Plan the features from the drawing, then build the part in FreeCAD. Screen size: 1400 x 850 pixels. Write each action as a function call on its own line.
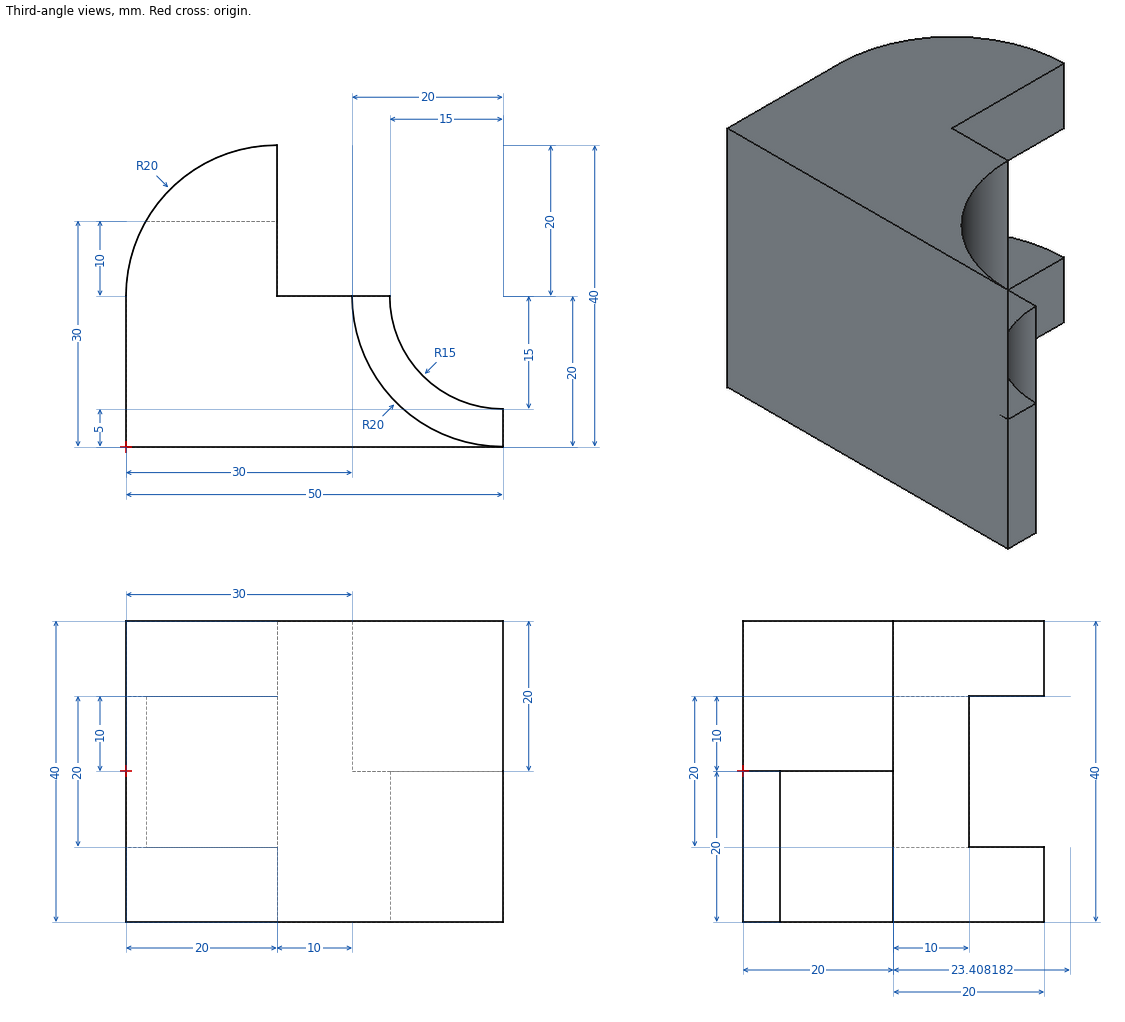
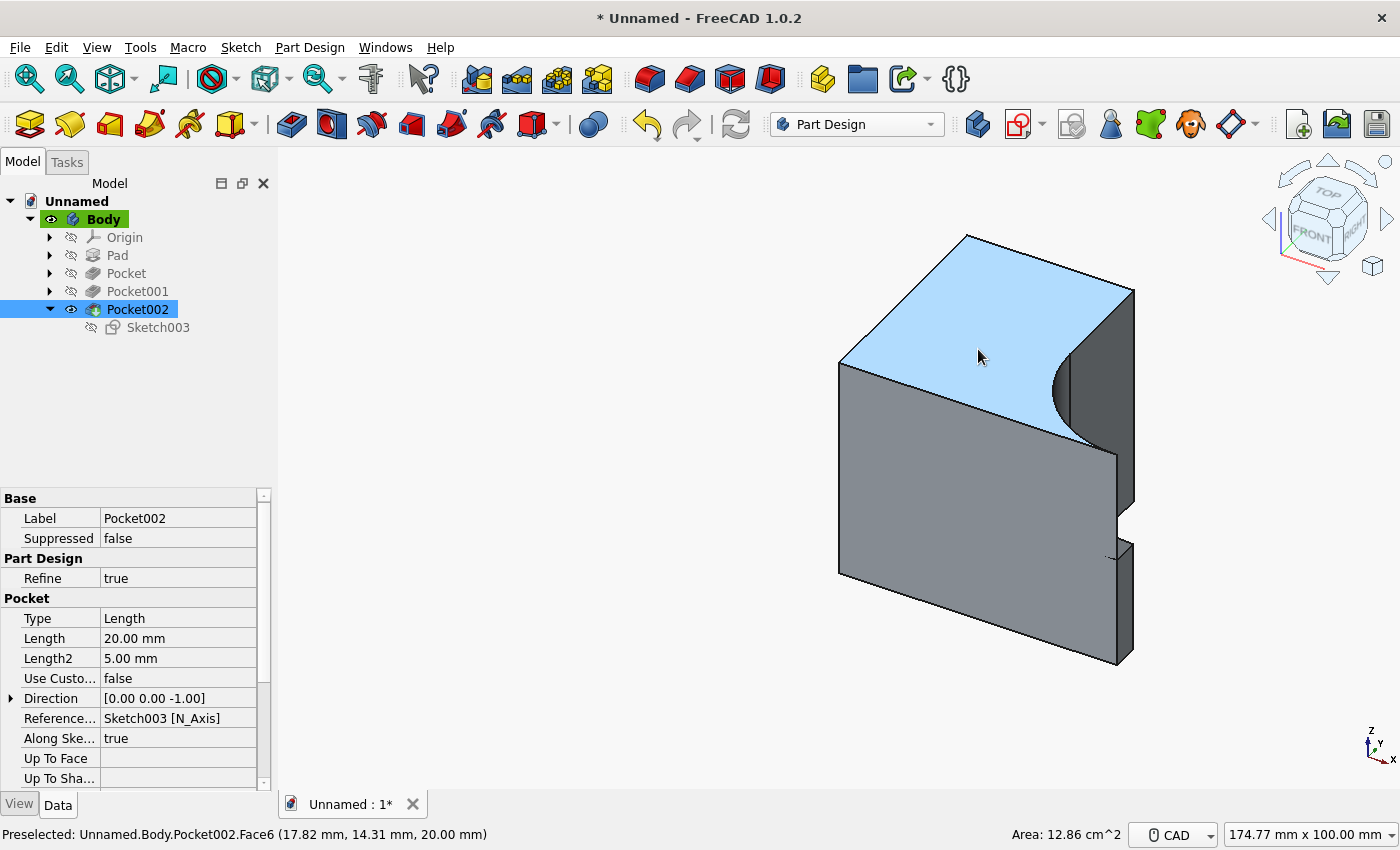
click(1018, 124)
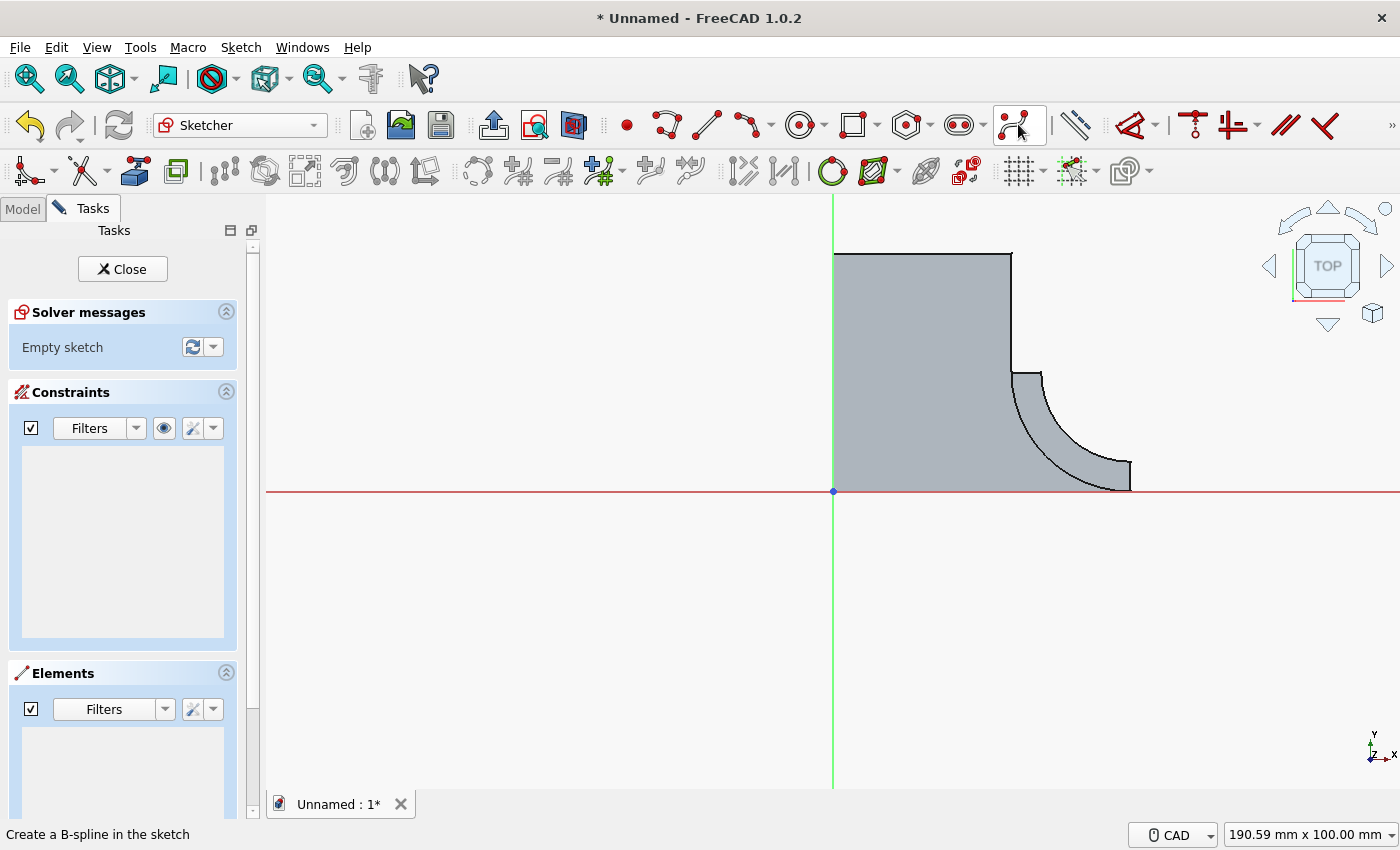
scroll(1153, 222, up, 2)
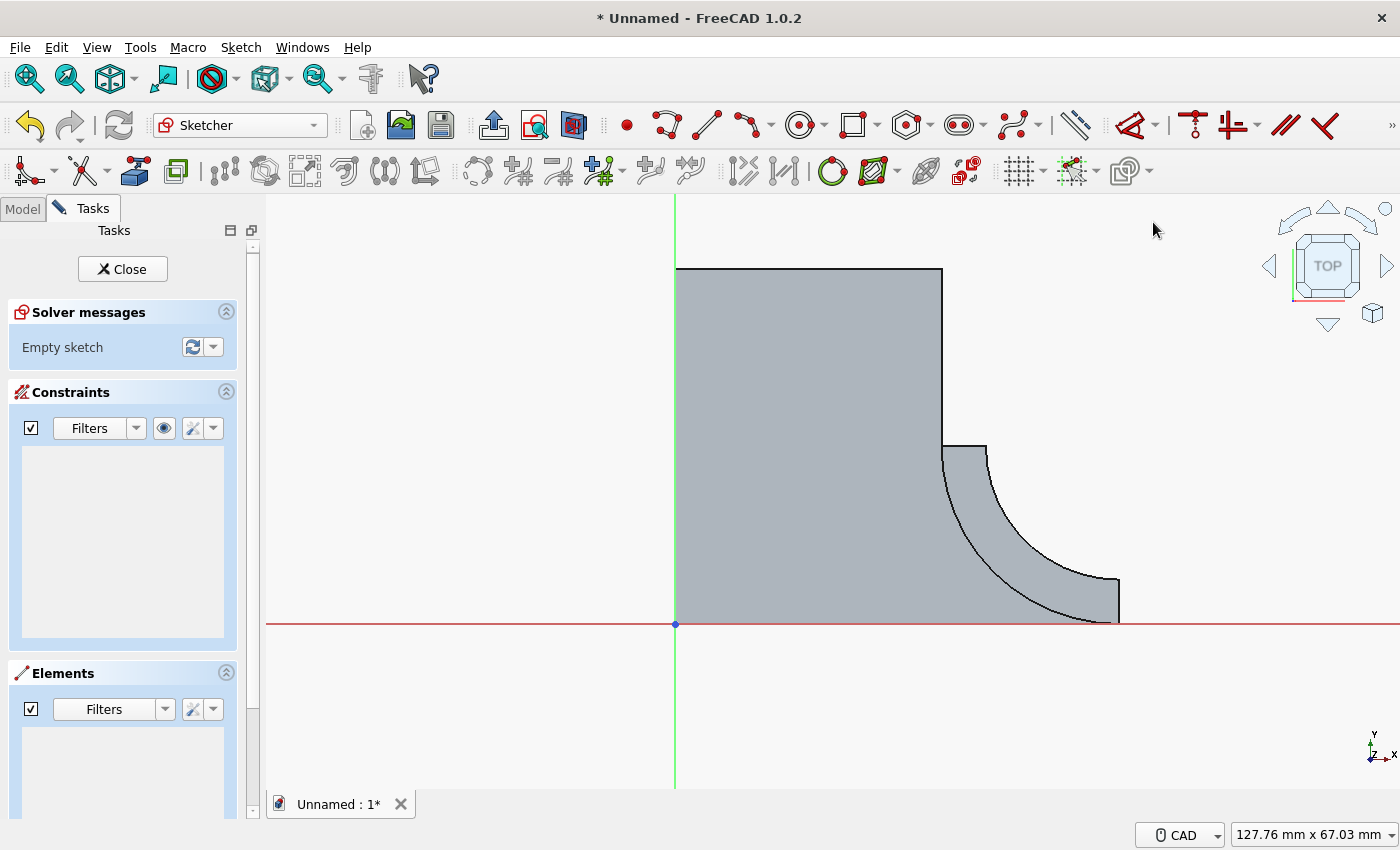
click(668, 126)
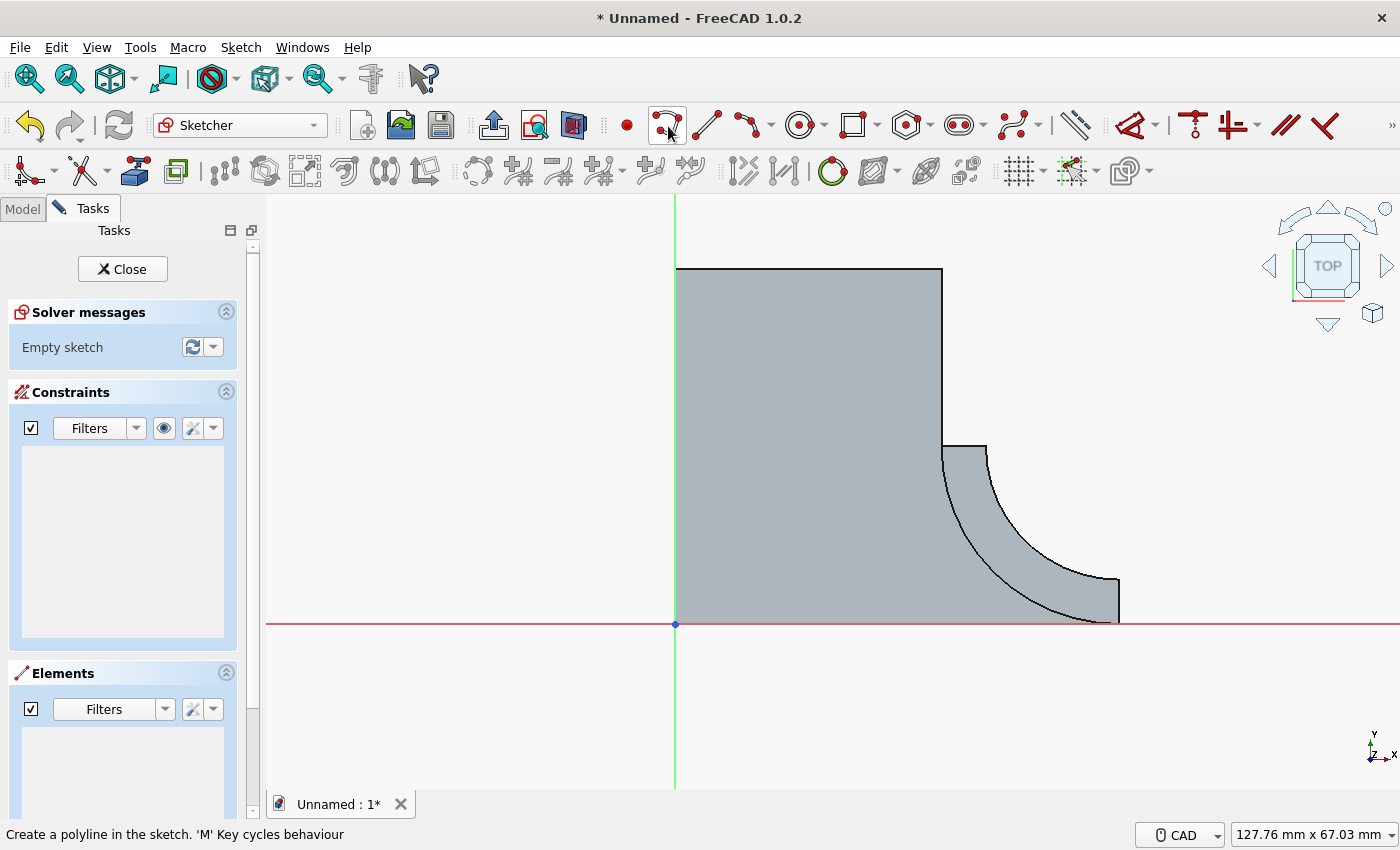
click(853, 269)
click(675, 269)
click(684, 446)
right_click(684, 446)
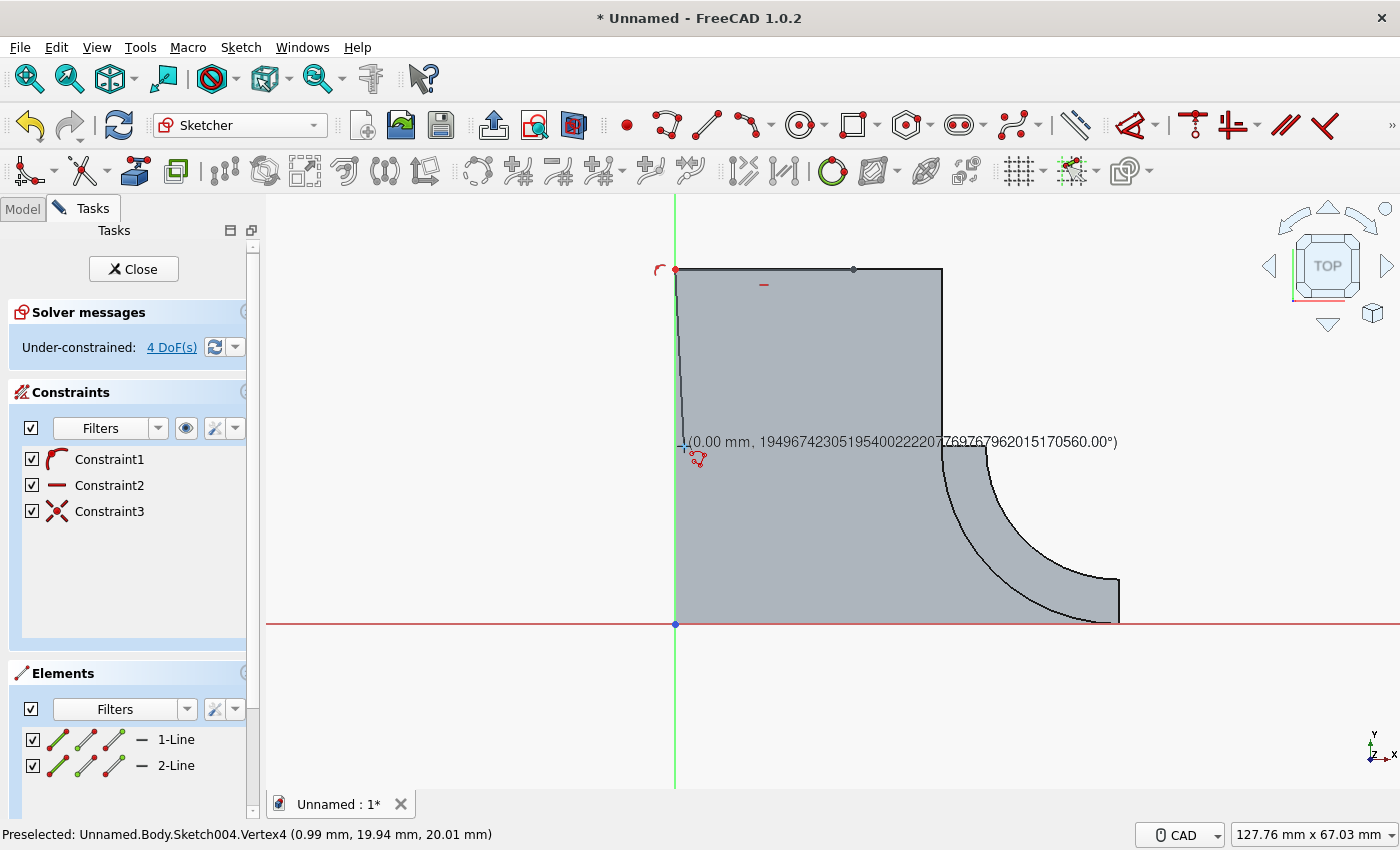
key(g)
key(3)
key(a)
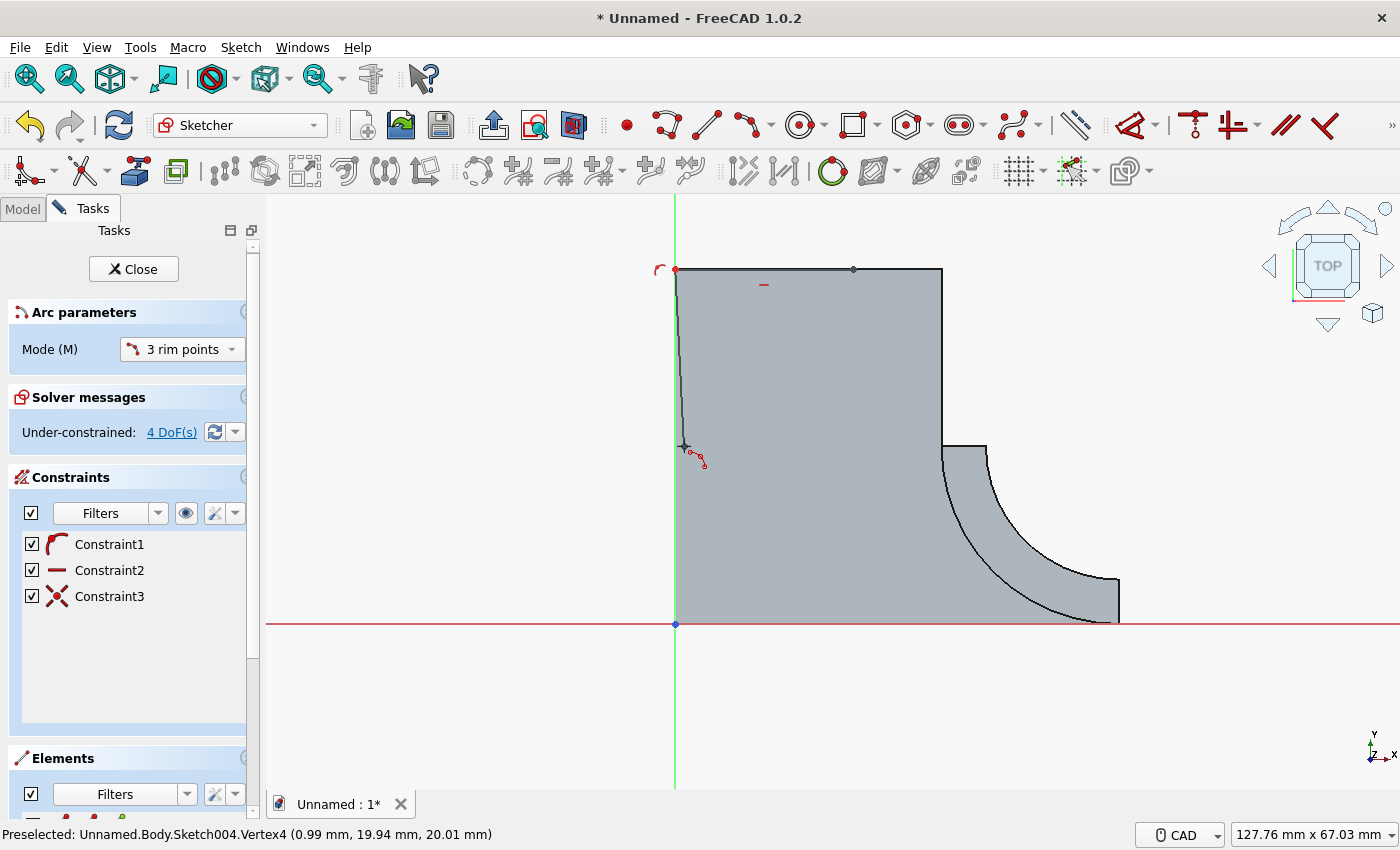
click(684, 447)
click(853, 270)
click(727, 321)
key(Escape)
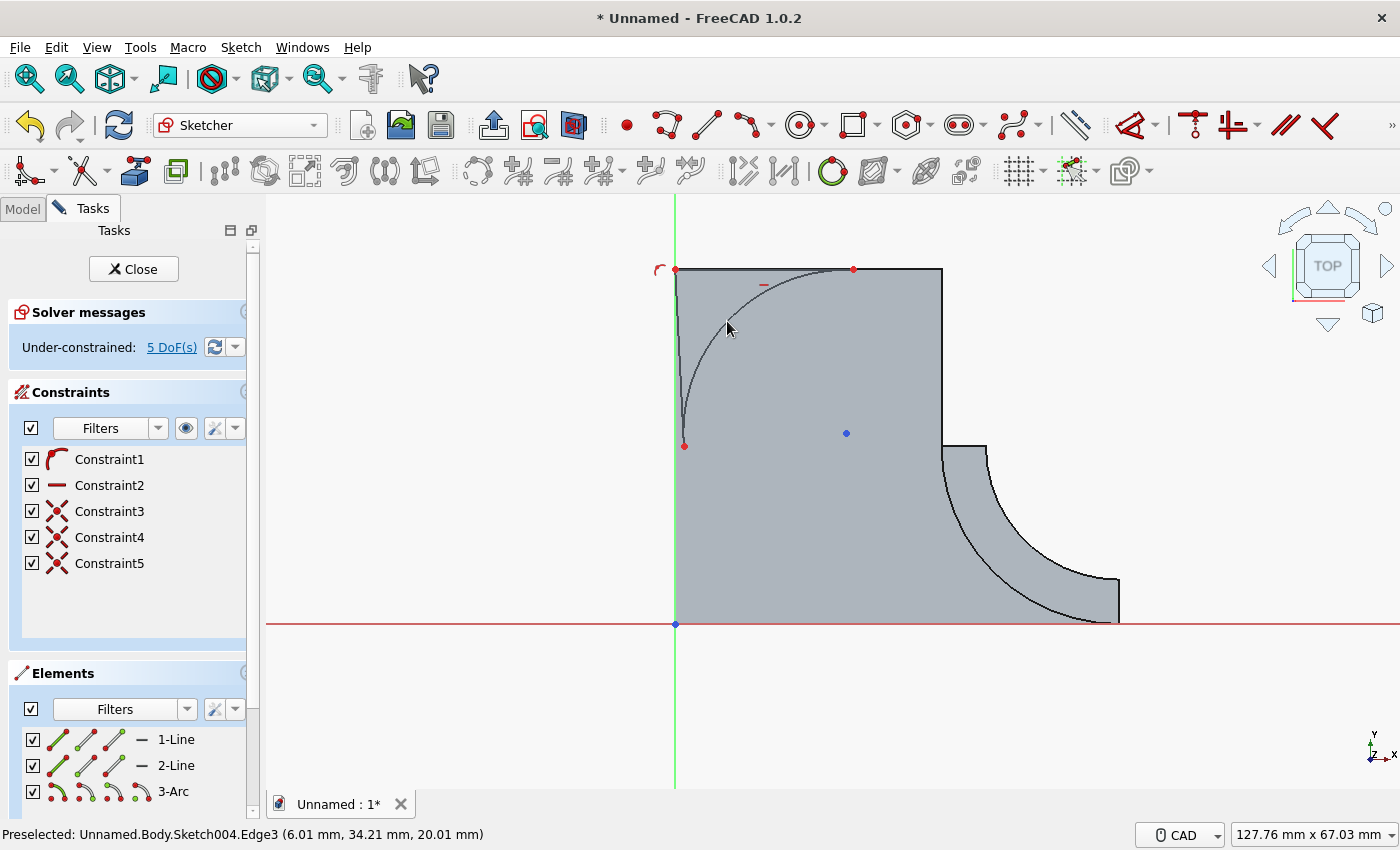
click(729, 270)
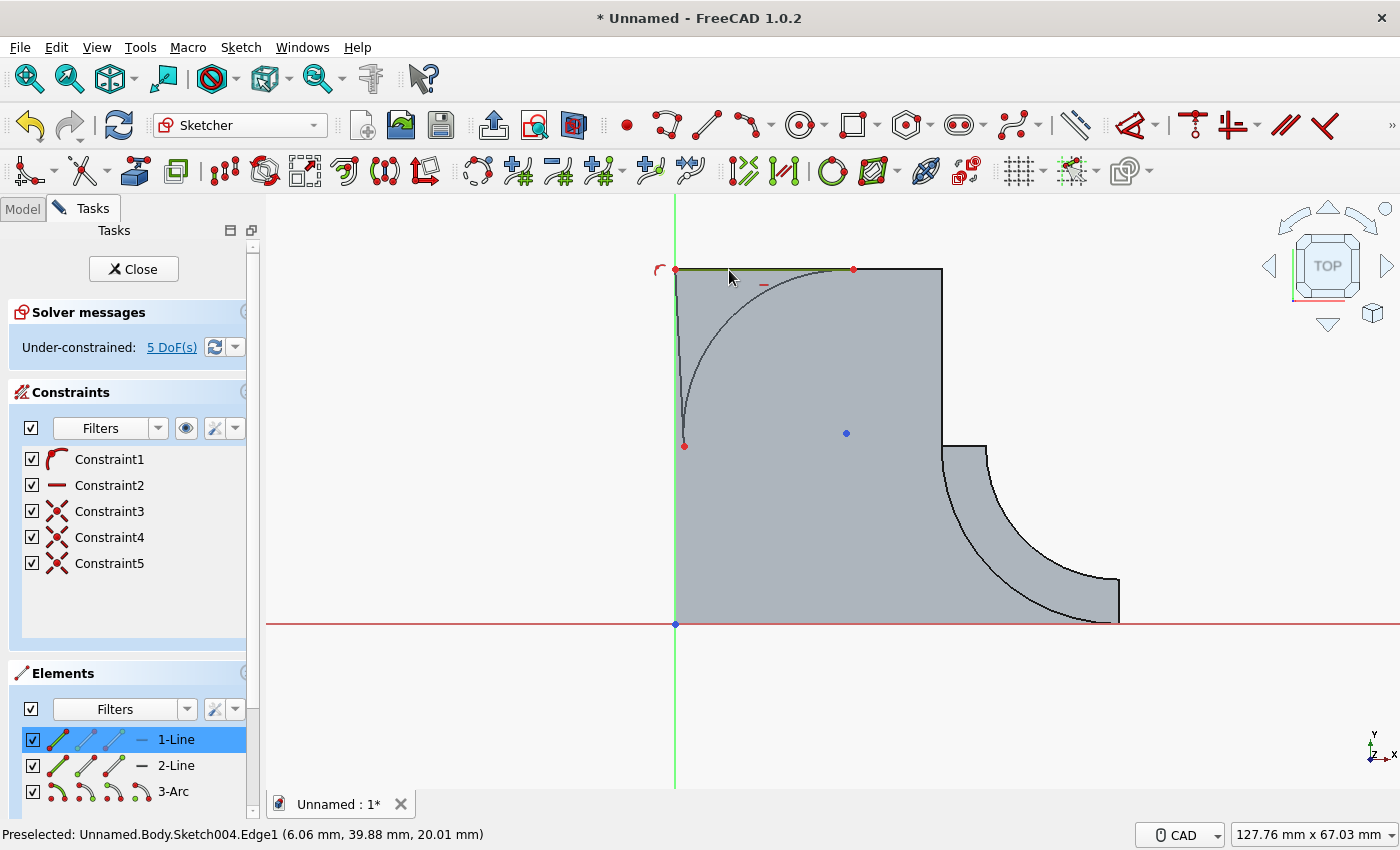
click(773, 288)